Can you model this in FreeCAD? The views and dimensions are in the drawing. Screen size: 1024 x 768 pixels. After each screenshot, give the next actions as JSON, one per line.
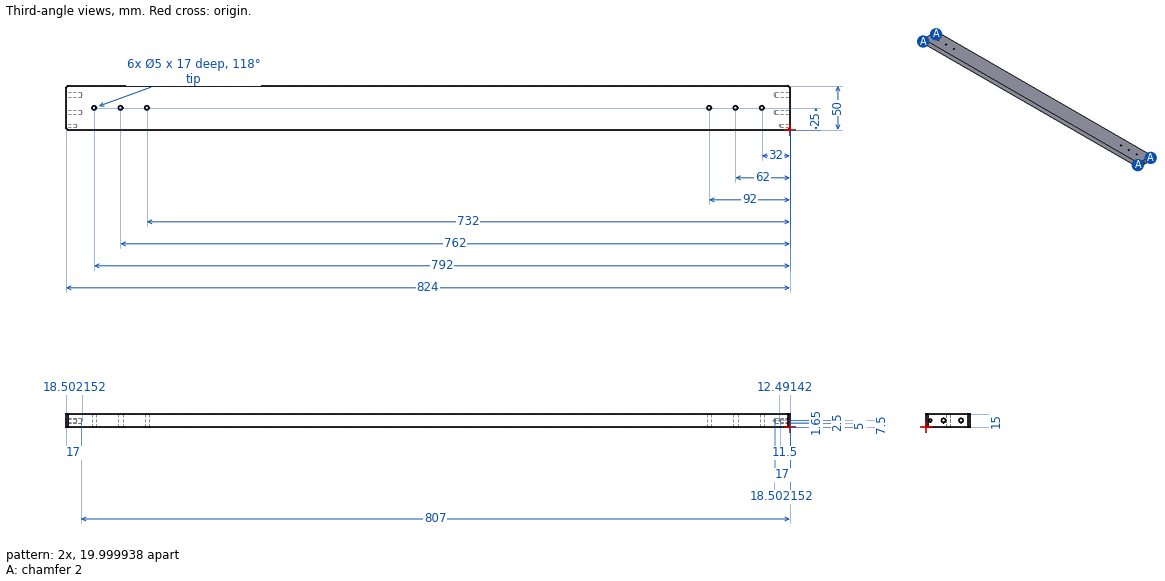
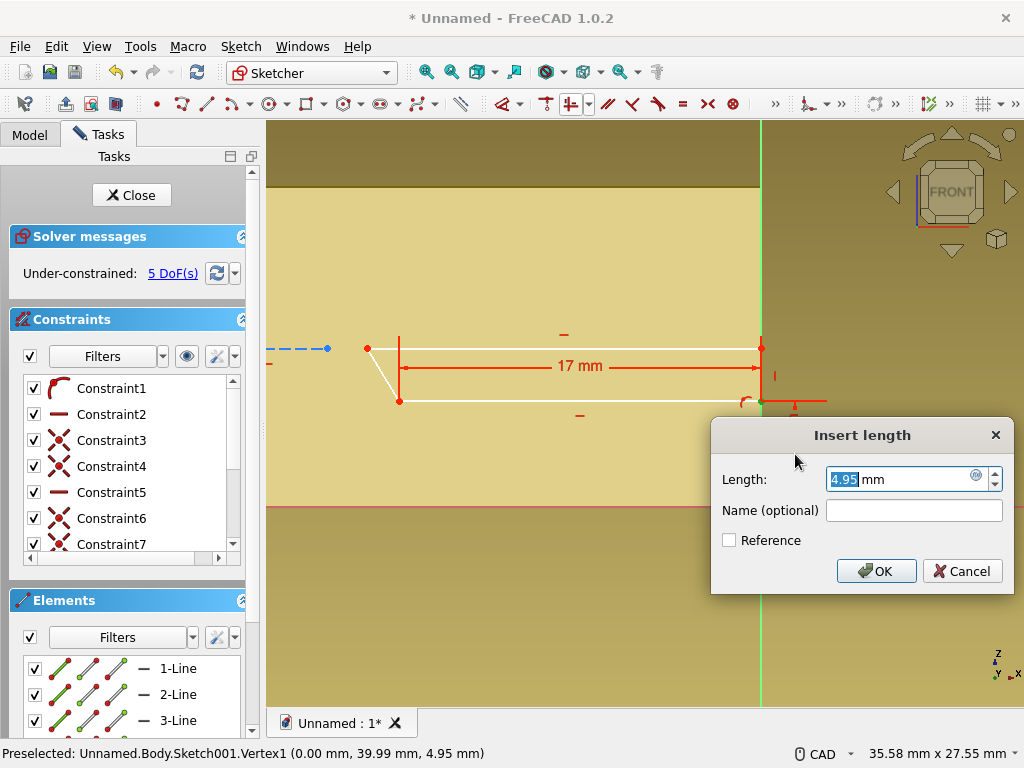
{"action": "type", "text": "5"}
{"action": "key", "text": "Return"}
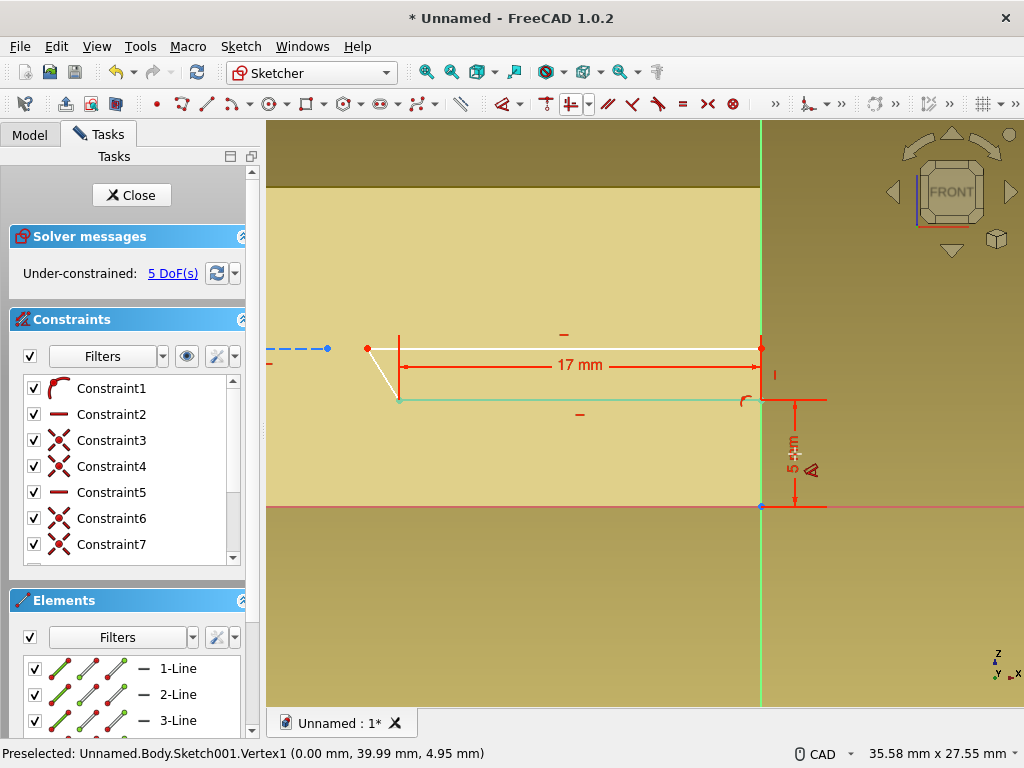
{"action": "left_click", "coordinate": [761, 364]}
{"action": "left_click", "coordinate": [795, 375]}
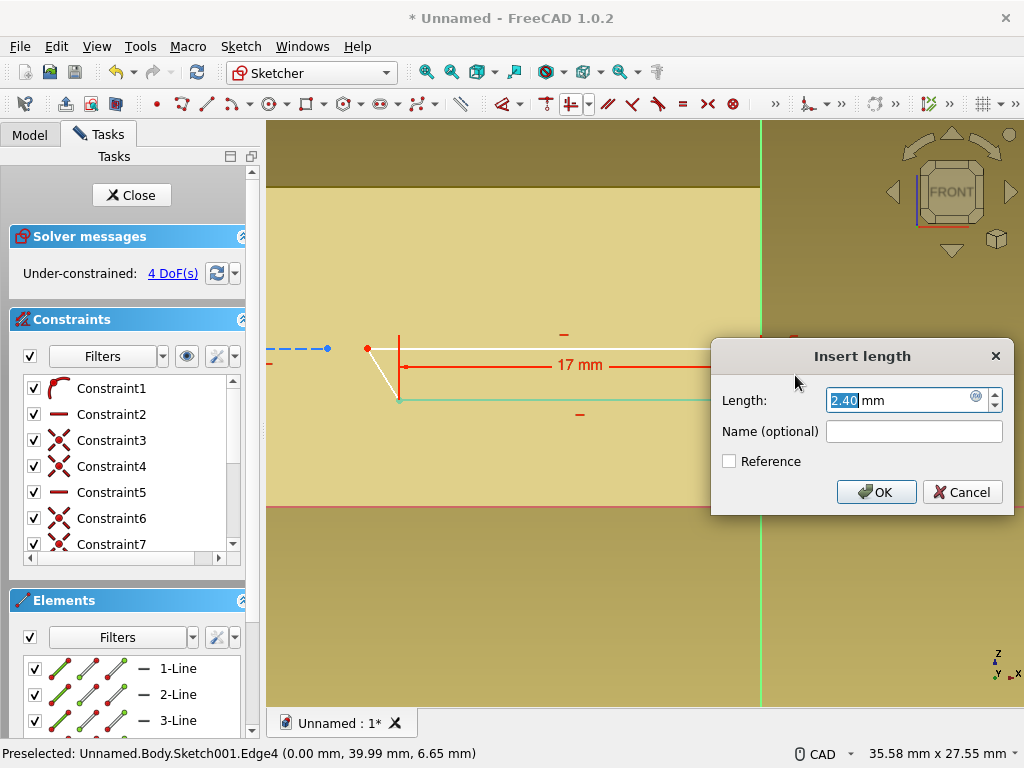
{"action": "type", "text": "2.5"}
{"action": "key", "text": "Return"}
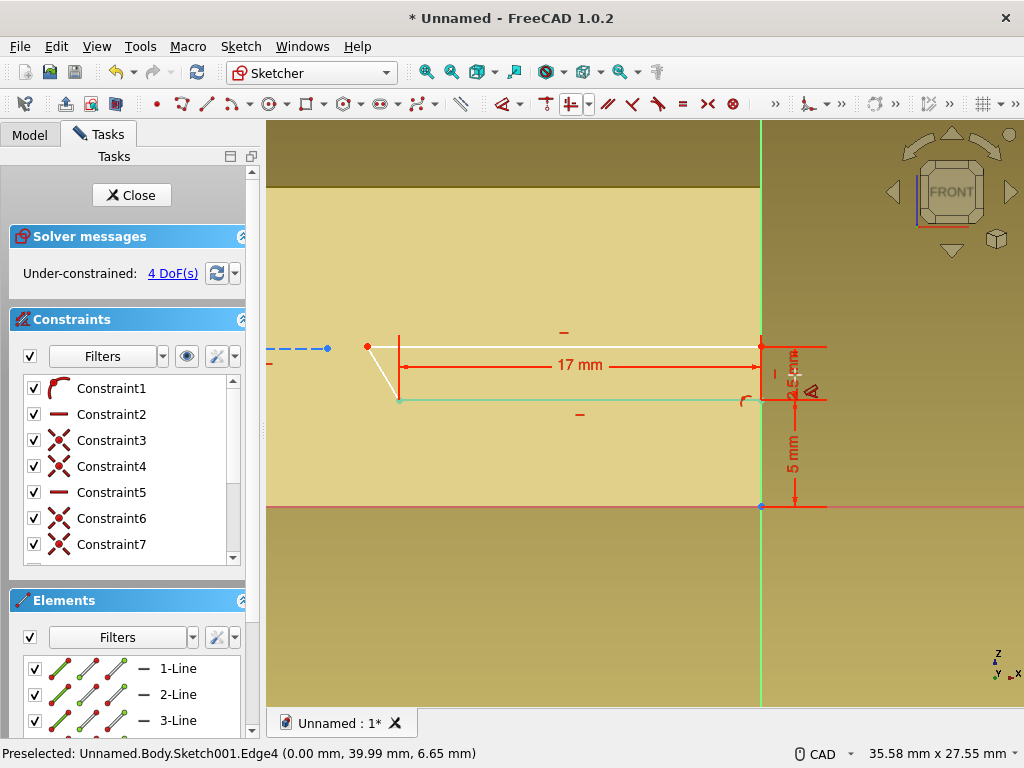
{"action": "left_click", "coordinate": [327, 349]}
{"action": "left_click", "coordinate": [795, 428]}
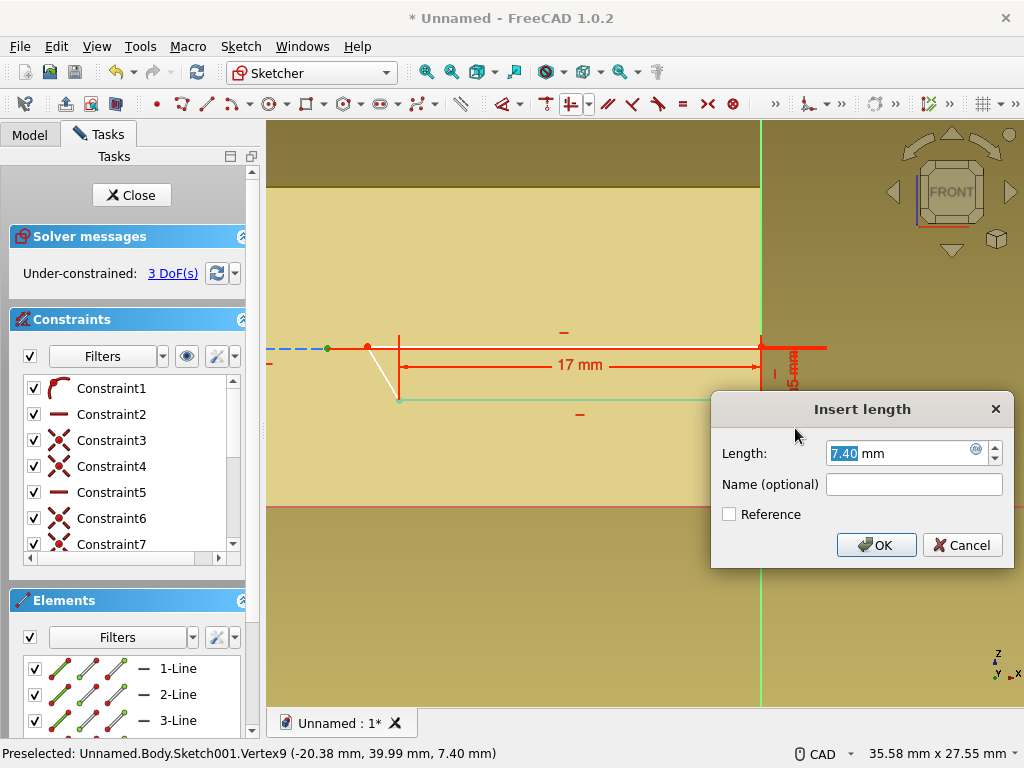
{"action": "type", "text": "7.5"}
{"action": "key", "text": "Return"}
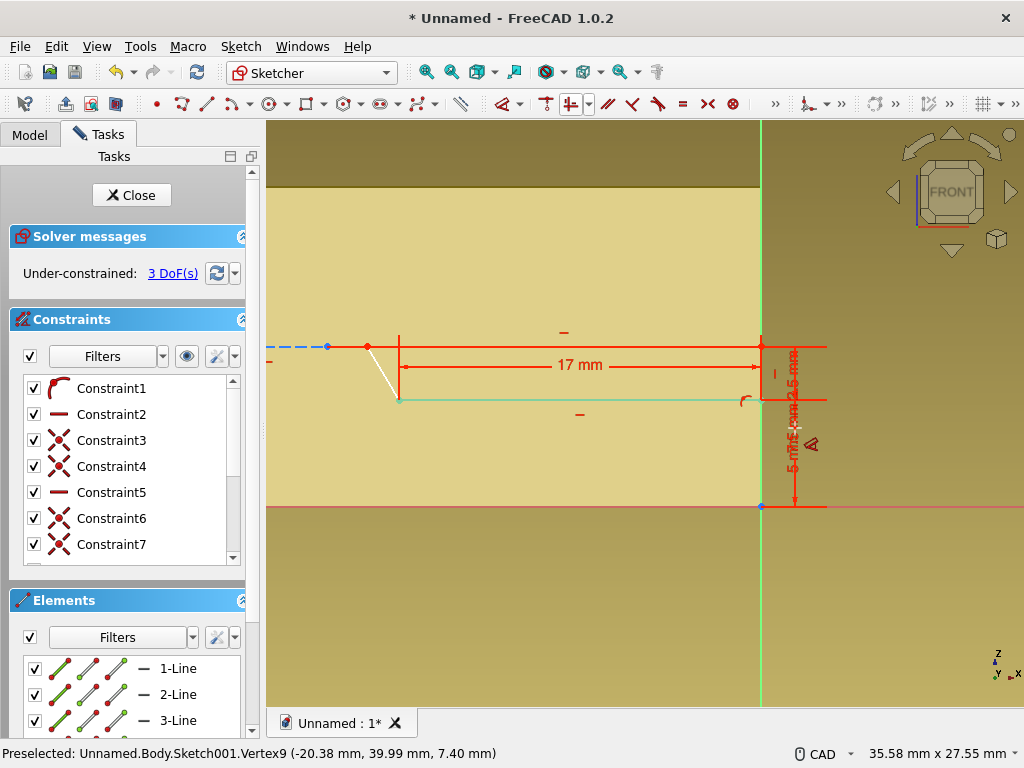
{"action": "left_click", "coordinate": [485, 347]}
{"action": "left_click", "coordinate": [564, 313]}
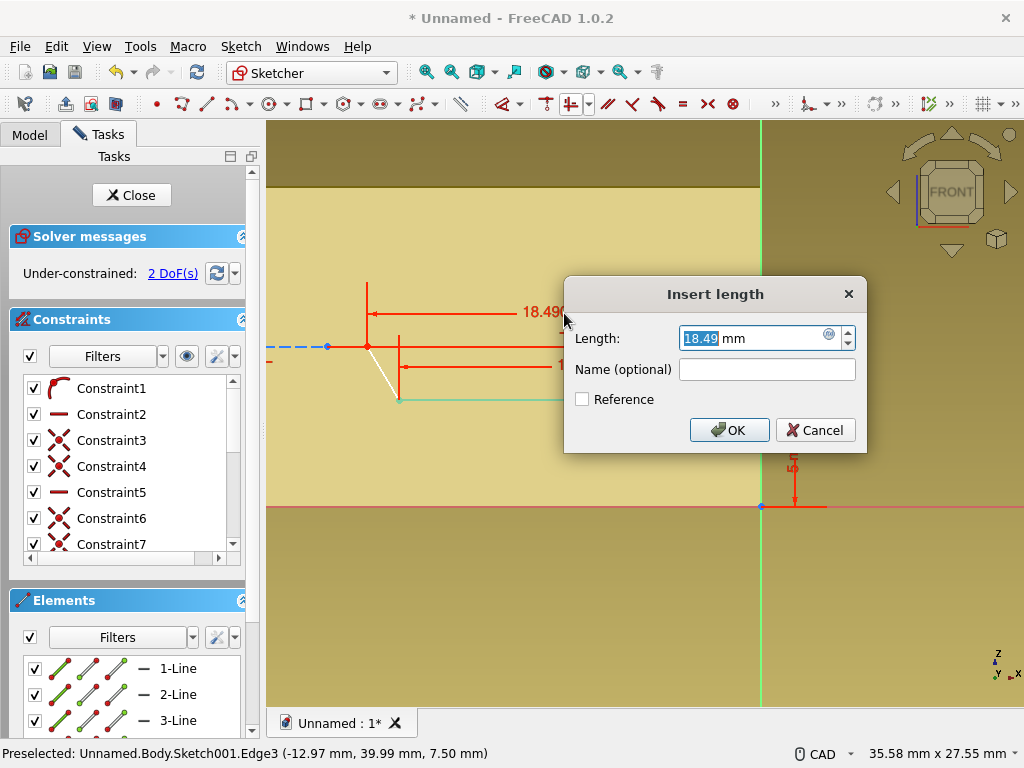
{"action": "type", "text": "18.502152"}
{"action": "key", "text": "Return"}
{"action": "key", "text": "Escape"}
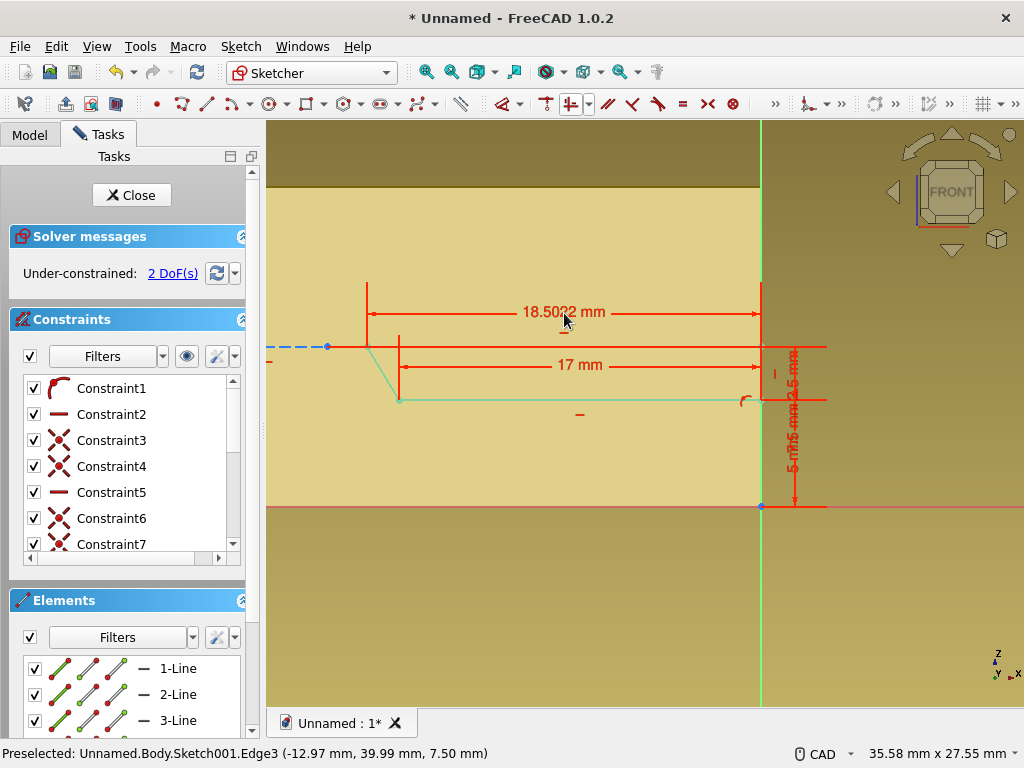
{"action": "left_click", "coordinate": [132, 195]}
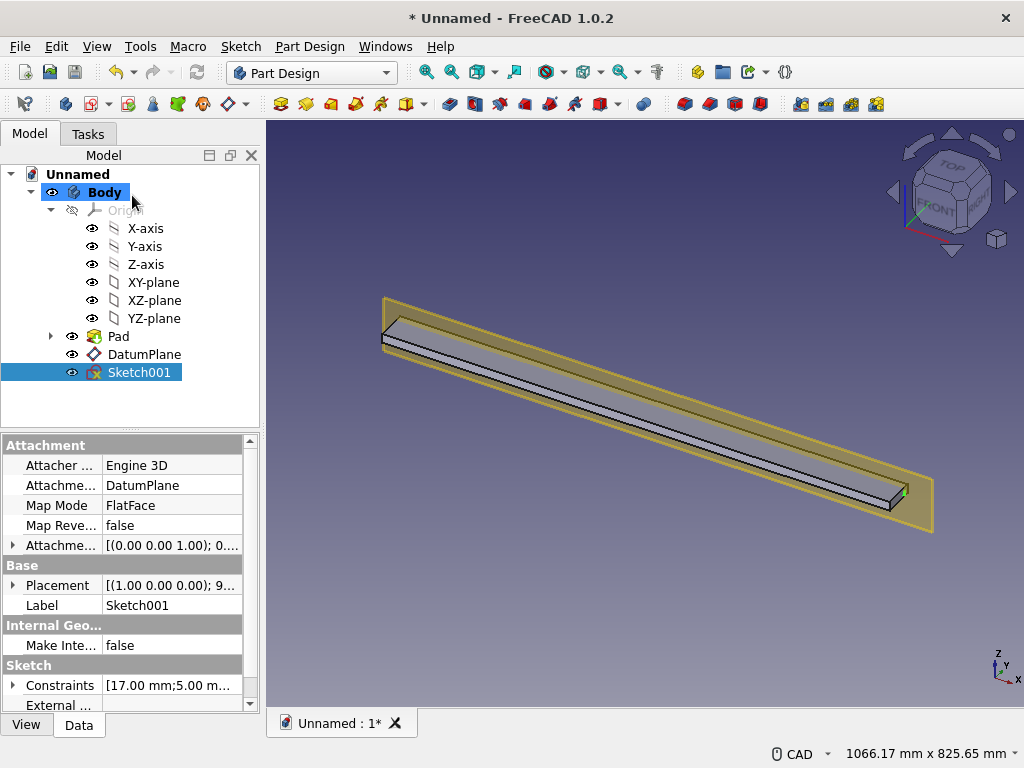
{"action": "left_click", "coordinate": [500, 104]}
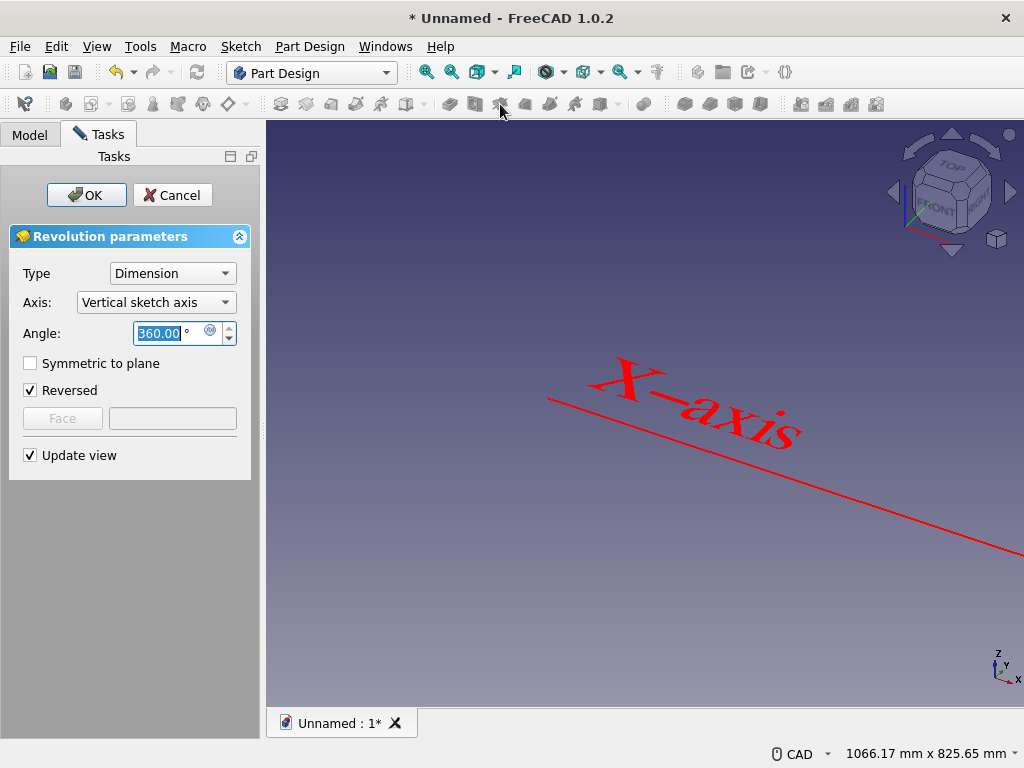
{"action": "left_click", "coordinate": [157, 302]}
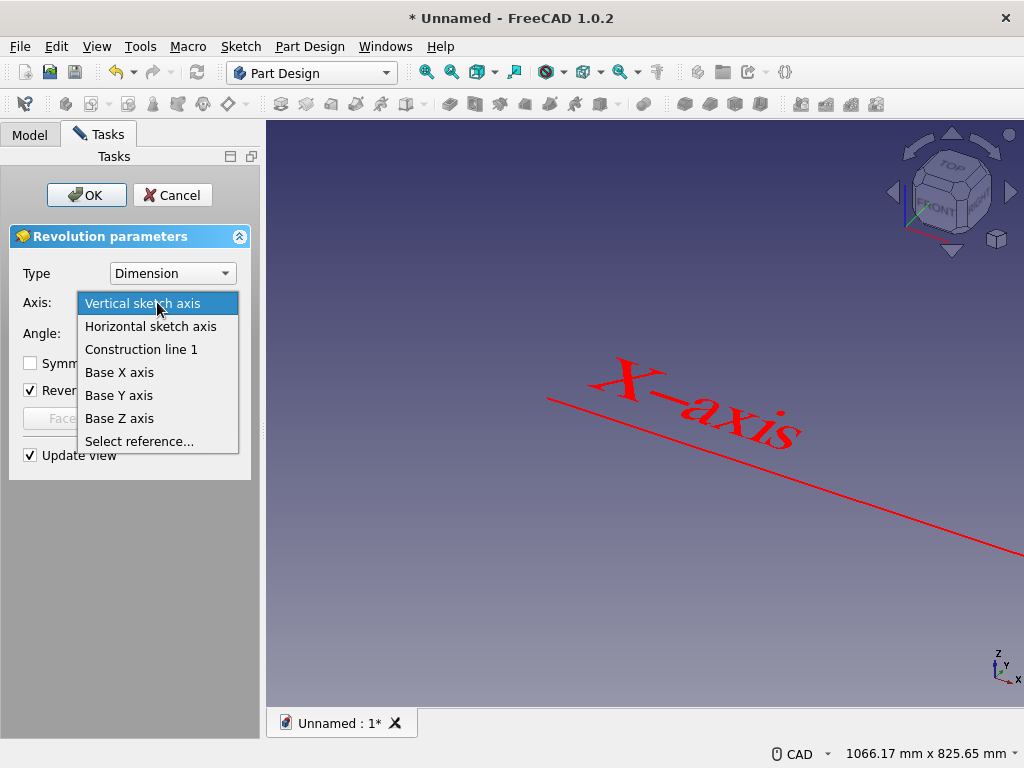
{"action": "left_click", "coordinate": [156, 350]}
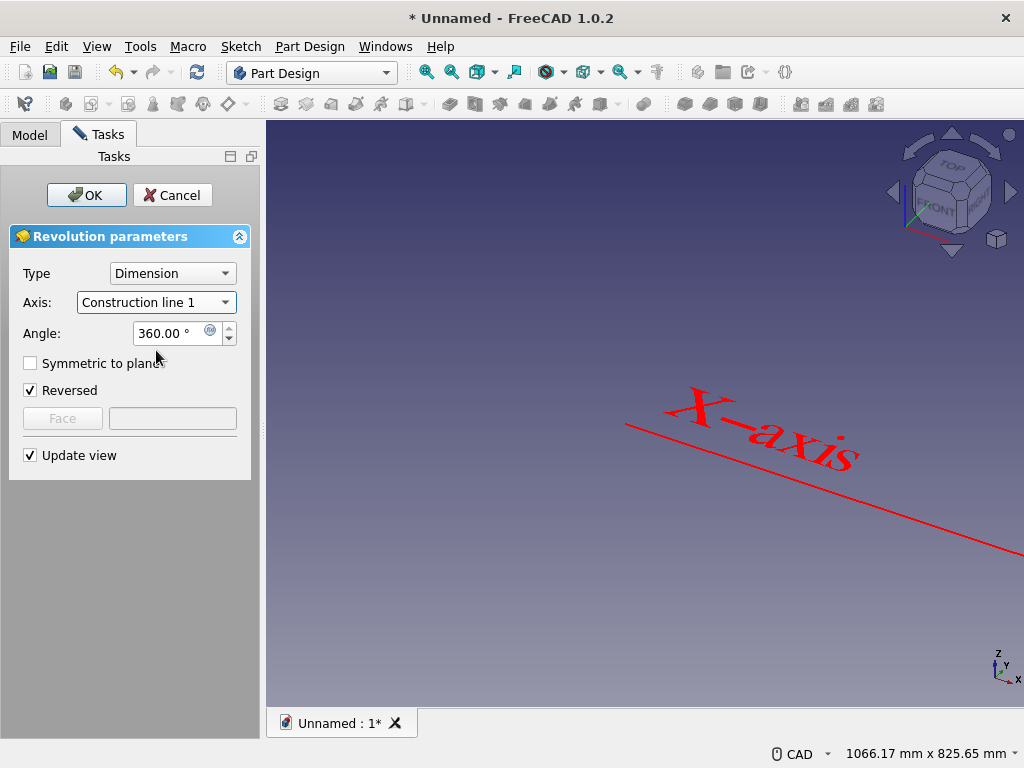
{"action": "left_click", "coordinate": [87, 195]}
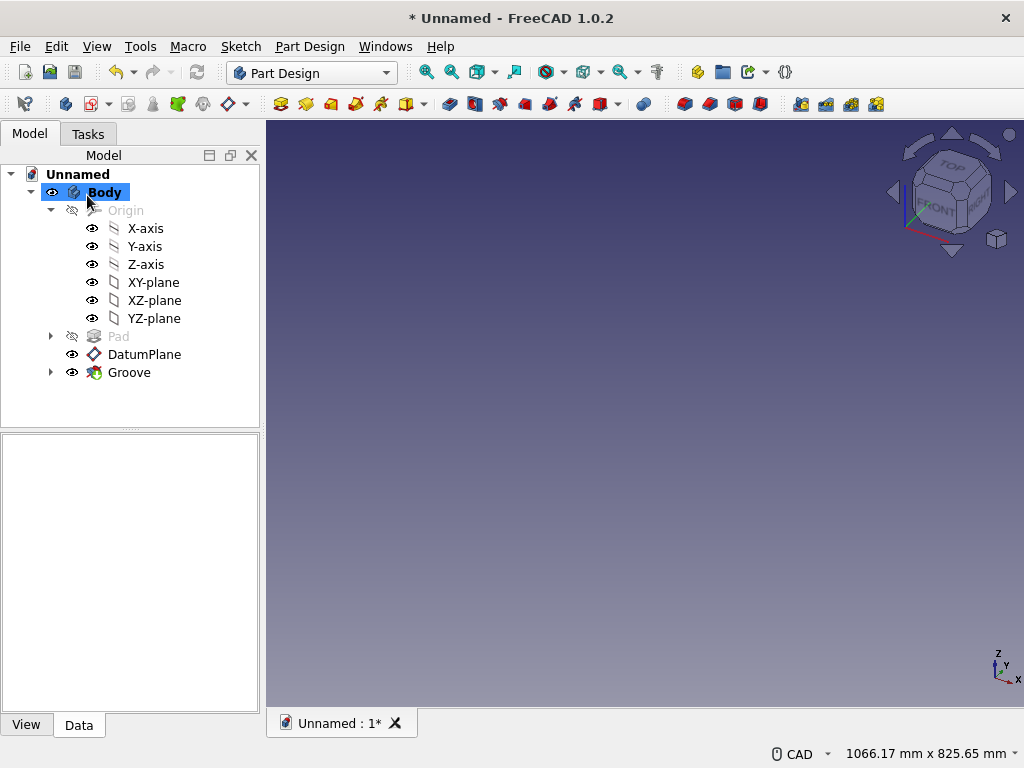
{"action": "left_click", "coordinate": [117, 354]}
{"action": "key", "text": "space"}